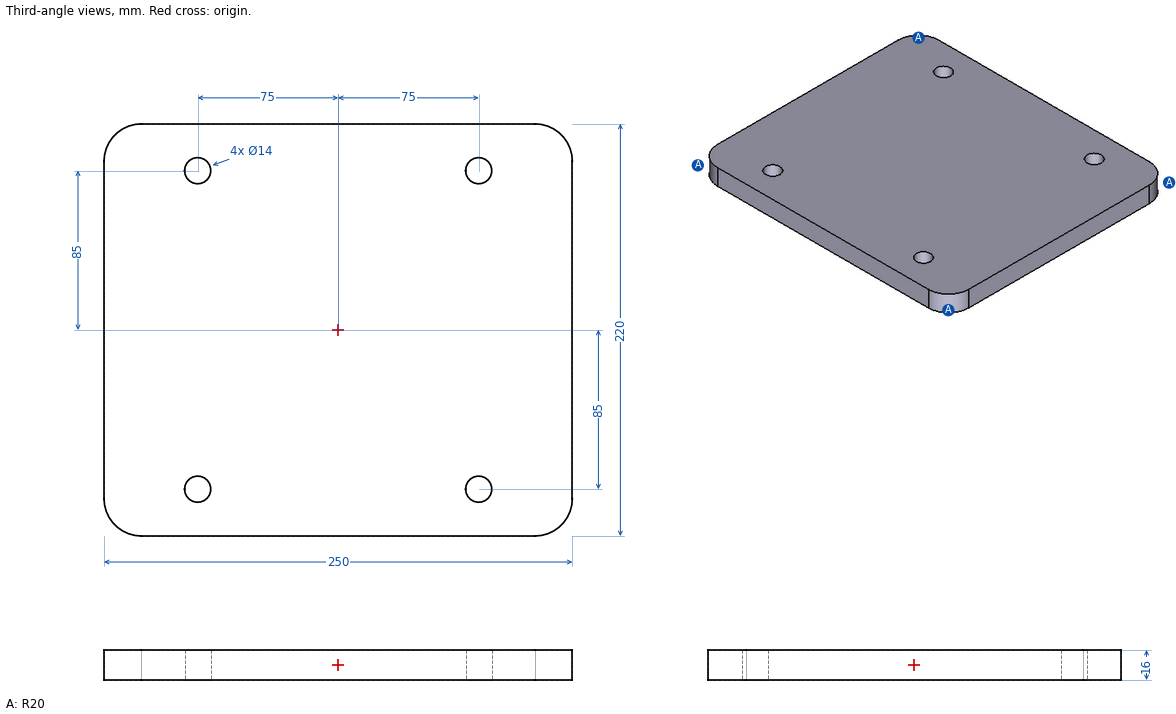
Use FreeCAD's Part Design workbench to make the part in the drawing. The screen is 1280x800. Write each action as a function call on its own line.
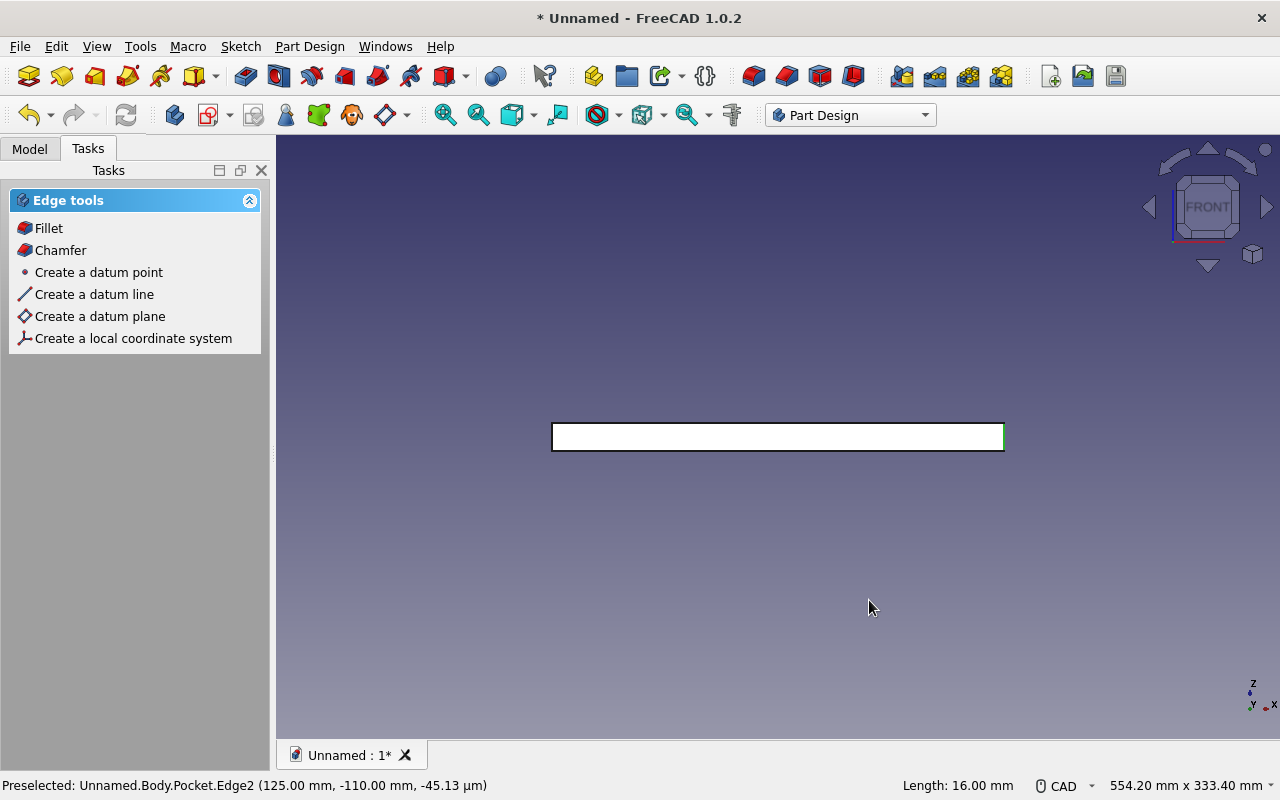
click(552, 436, ctrl)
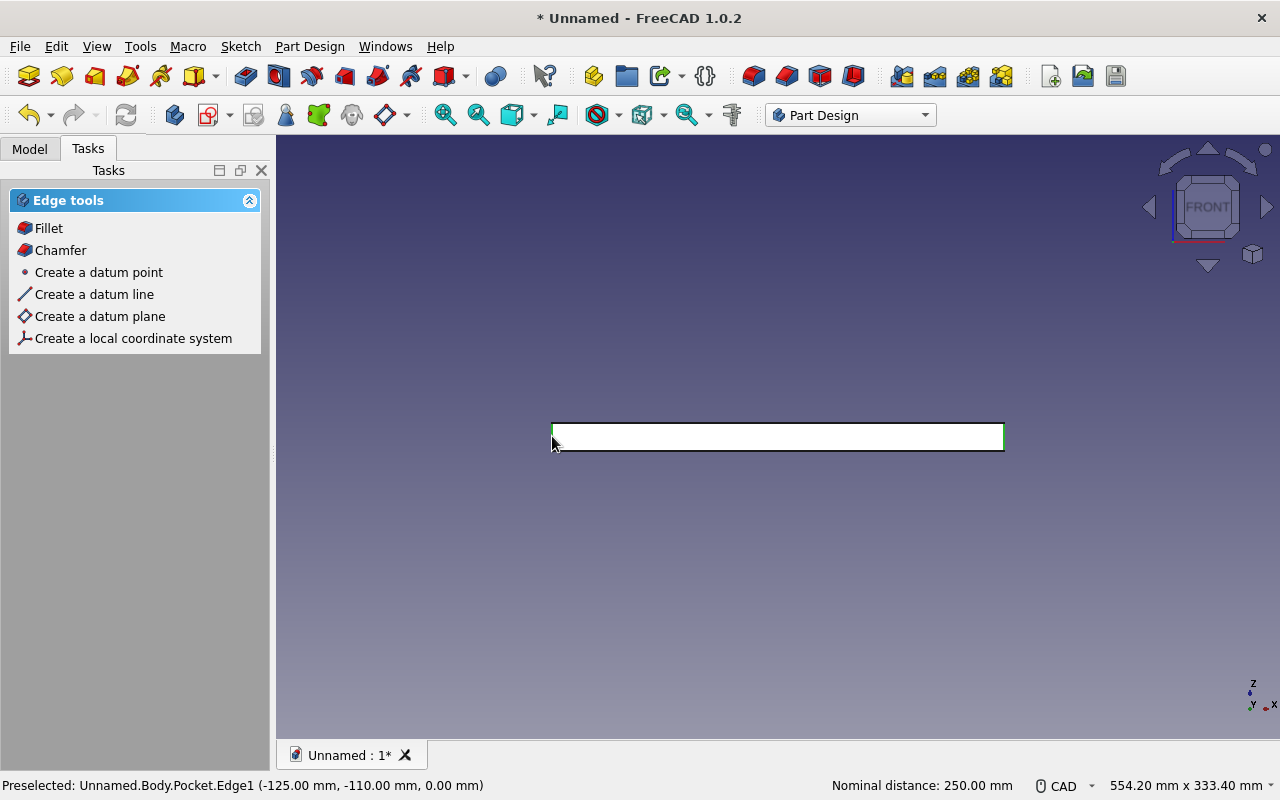
key(3)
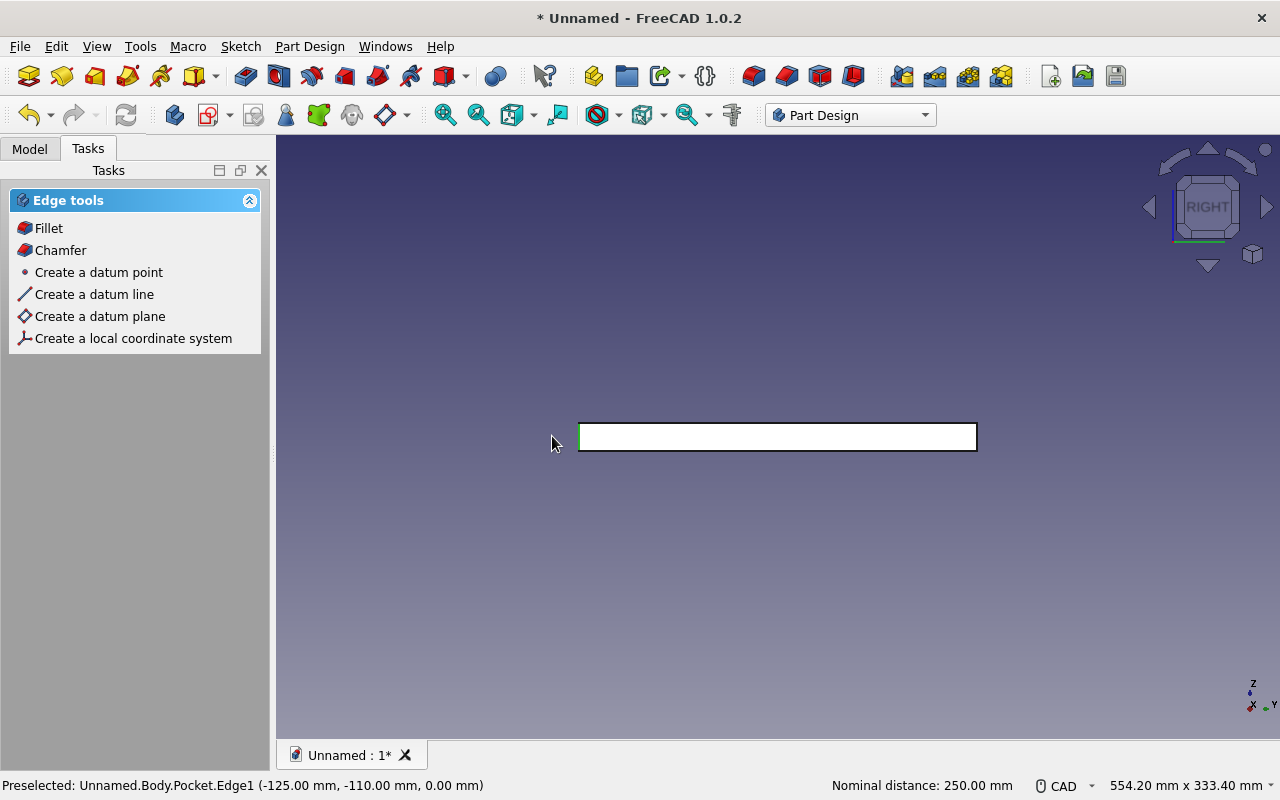
click(446, 116)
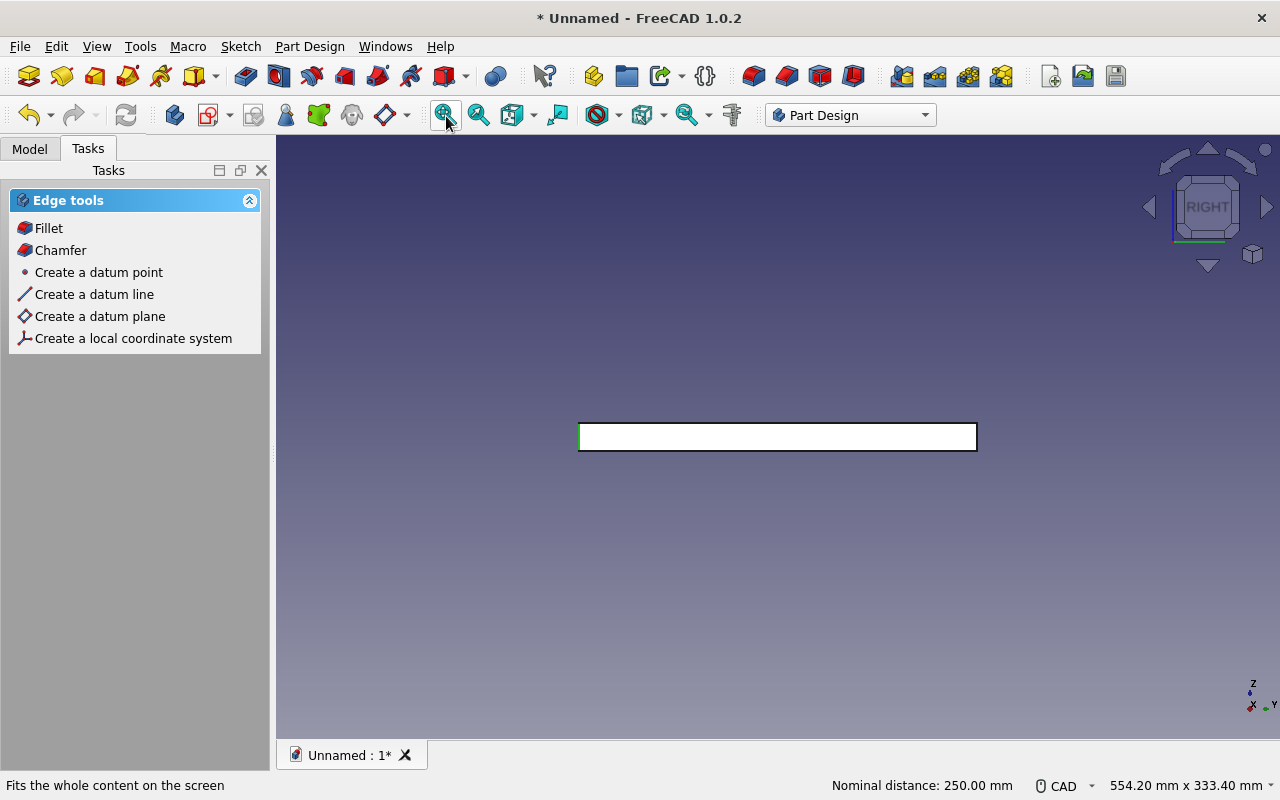
click(977, 436, ctrl)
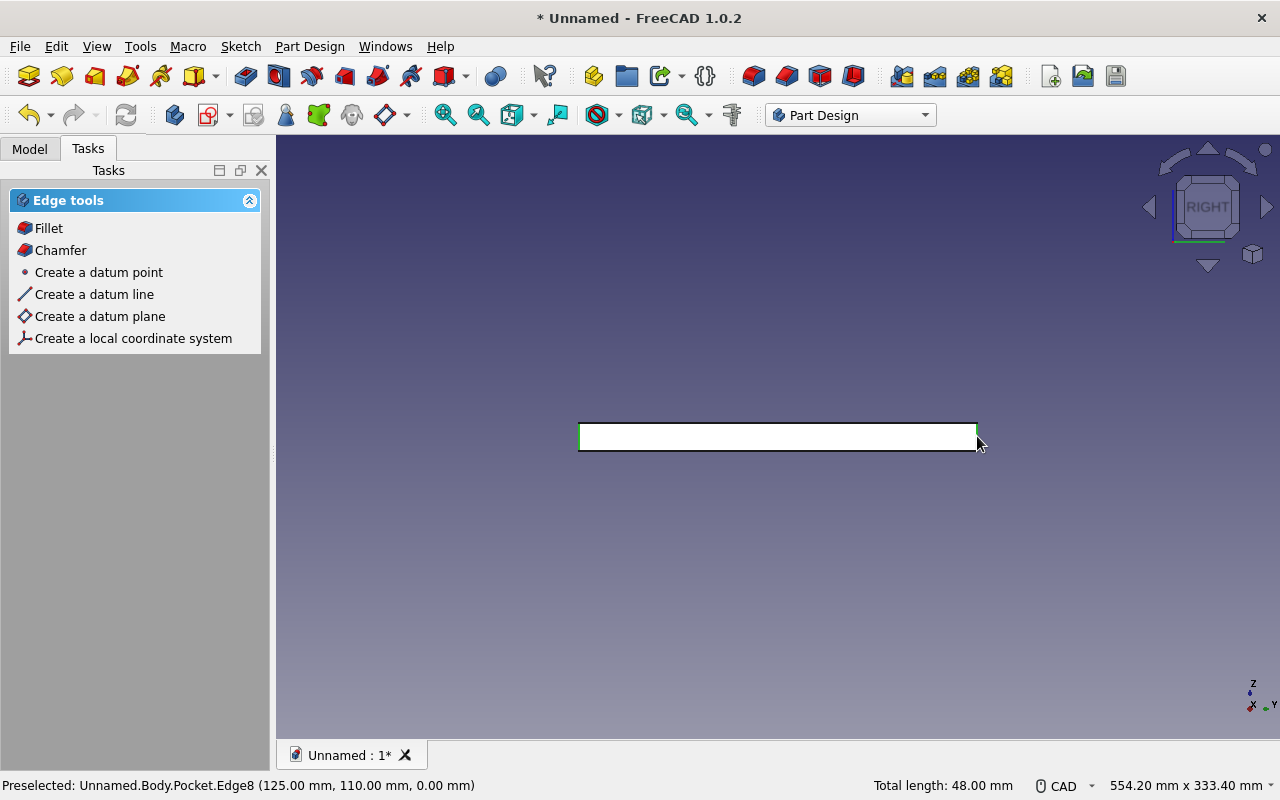
key(5)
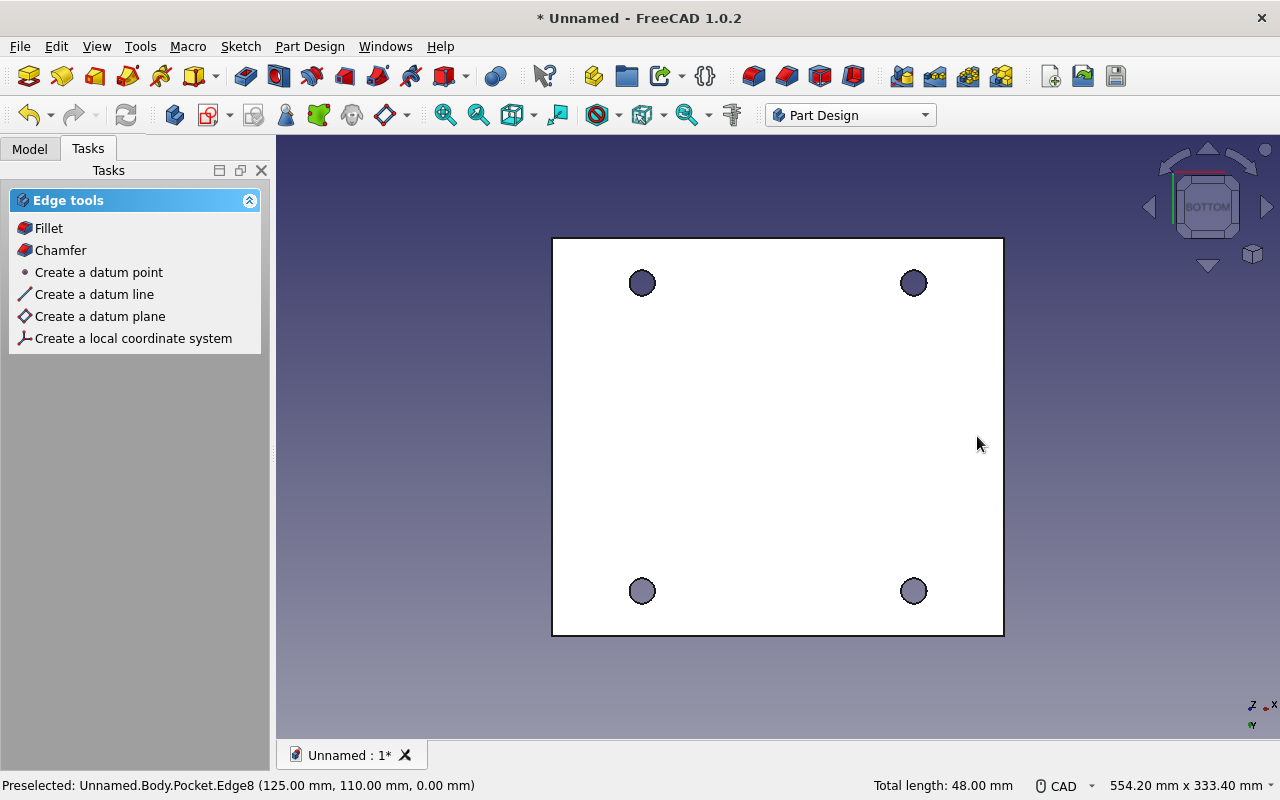
key(4)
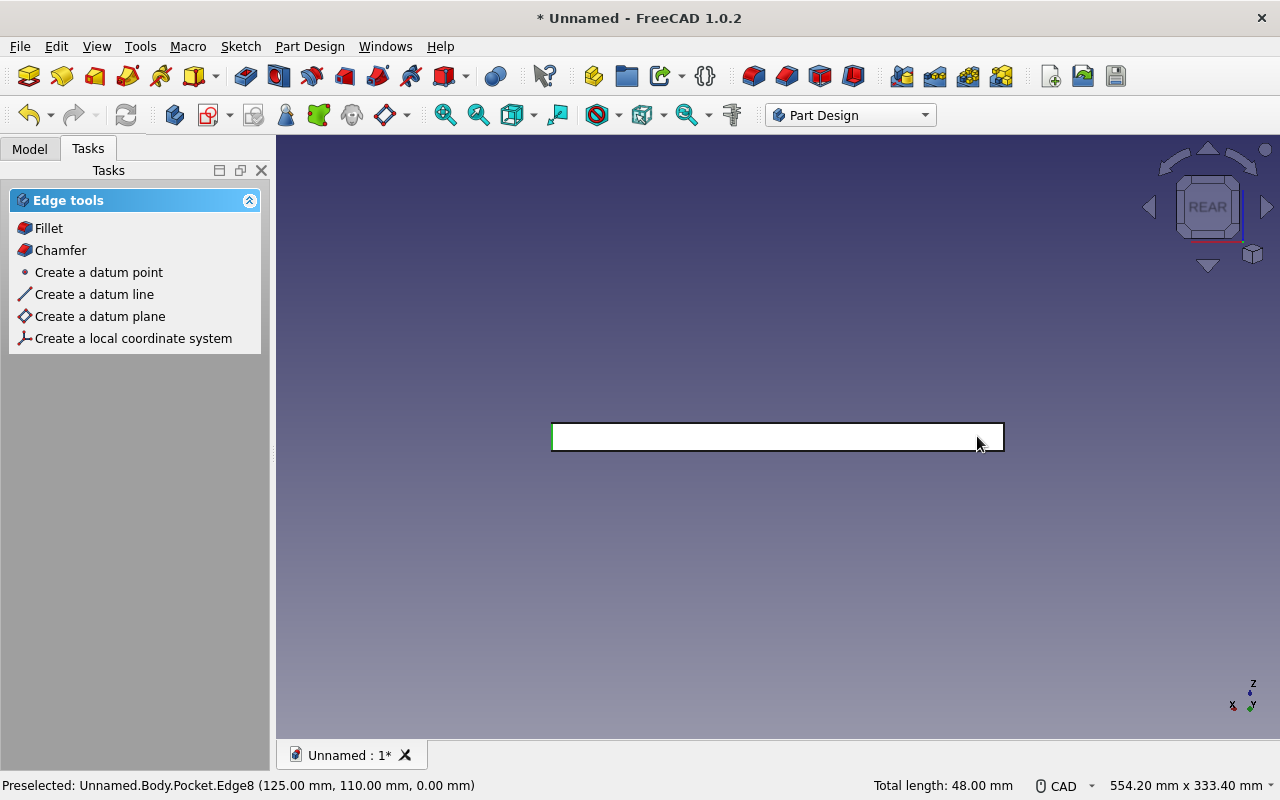
click(1004, 436, ctrl)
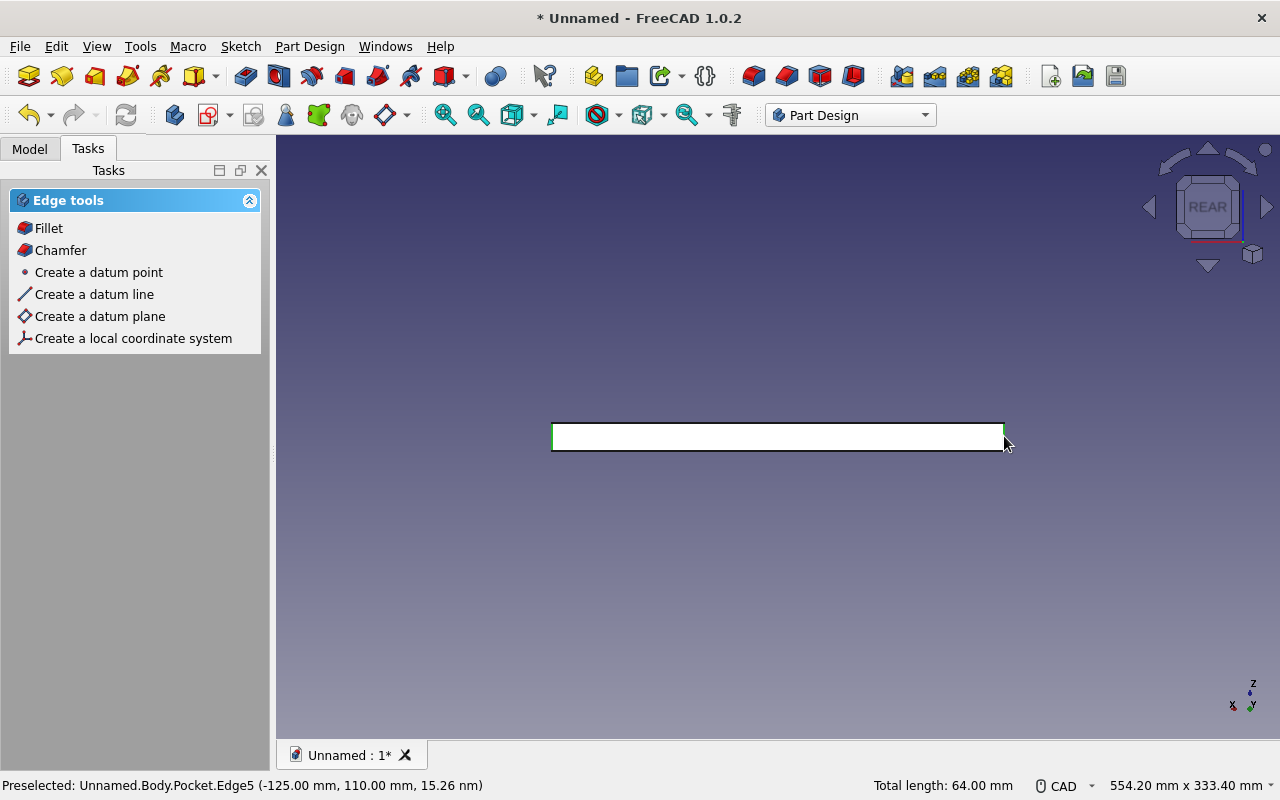
click(754, 76)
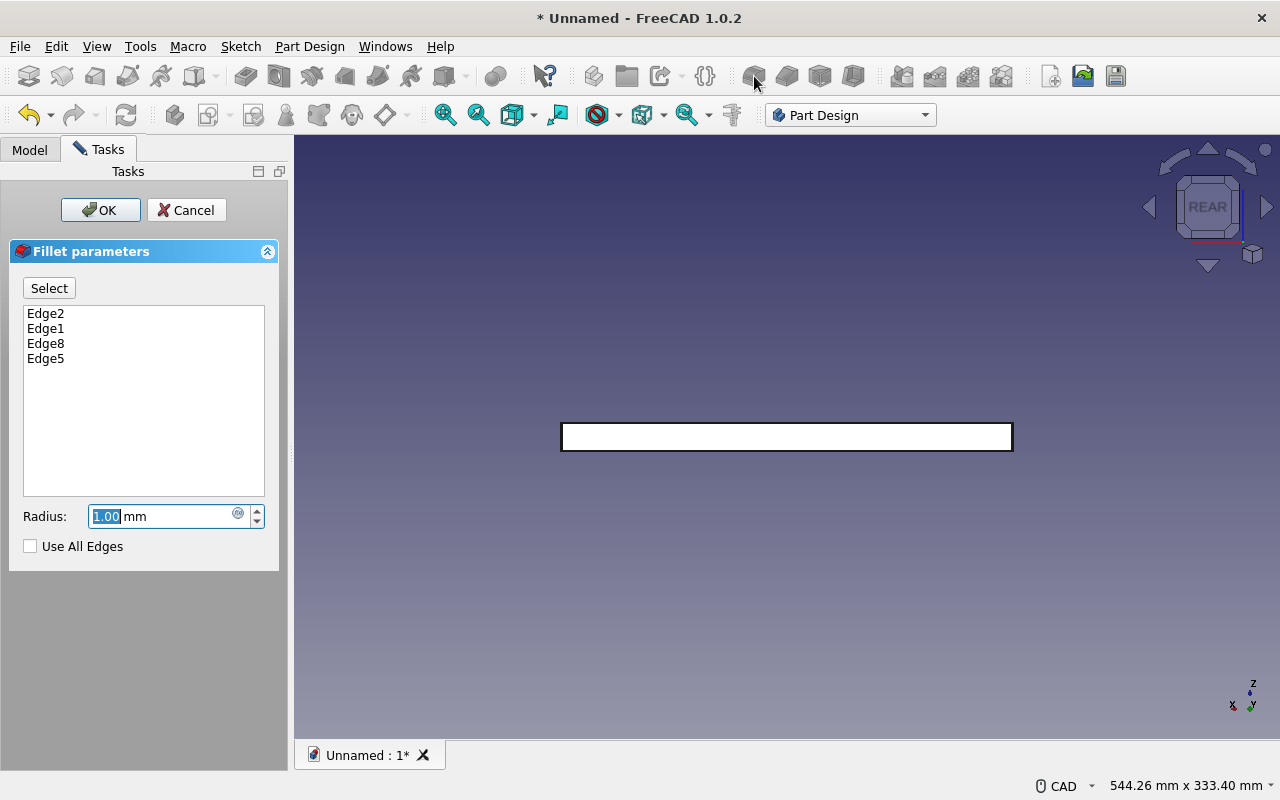
text(20)
key(Tab)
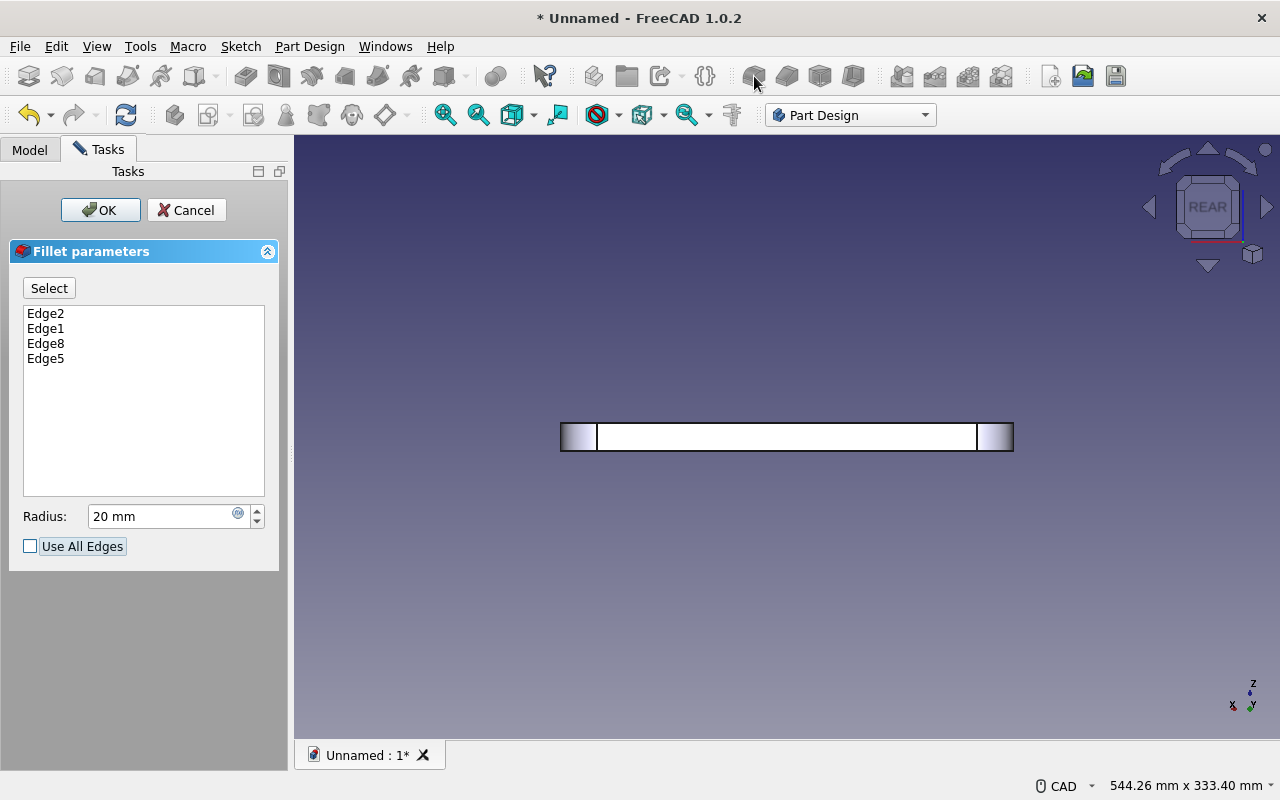
click(101, 210)